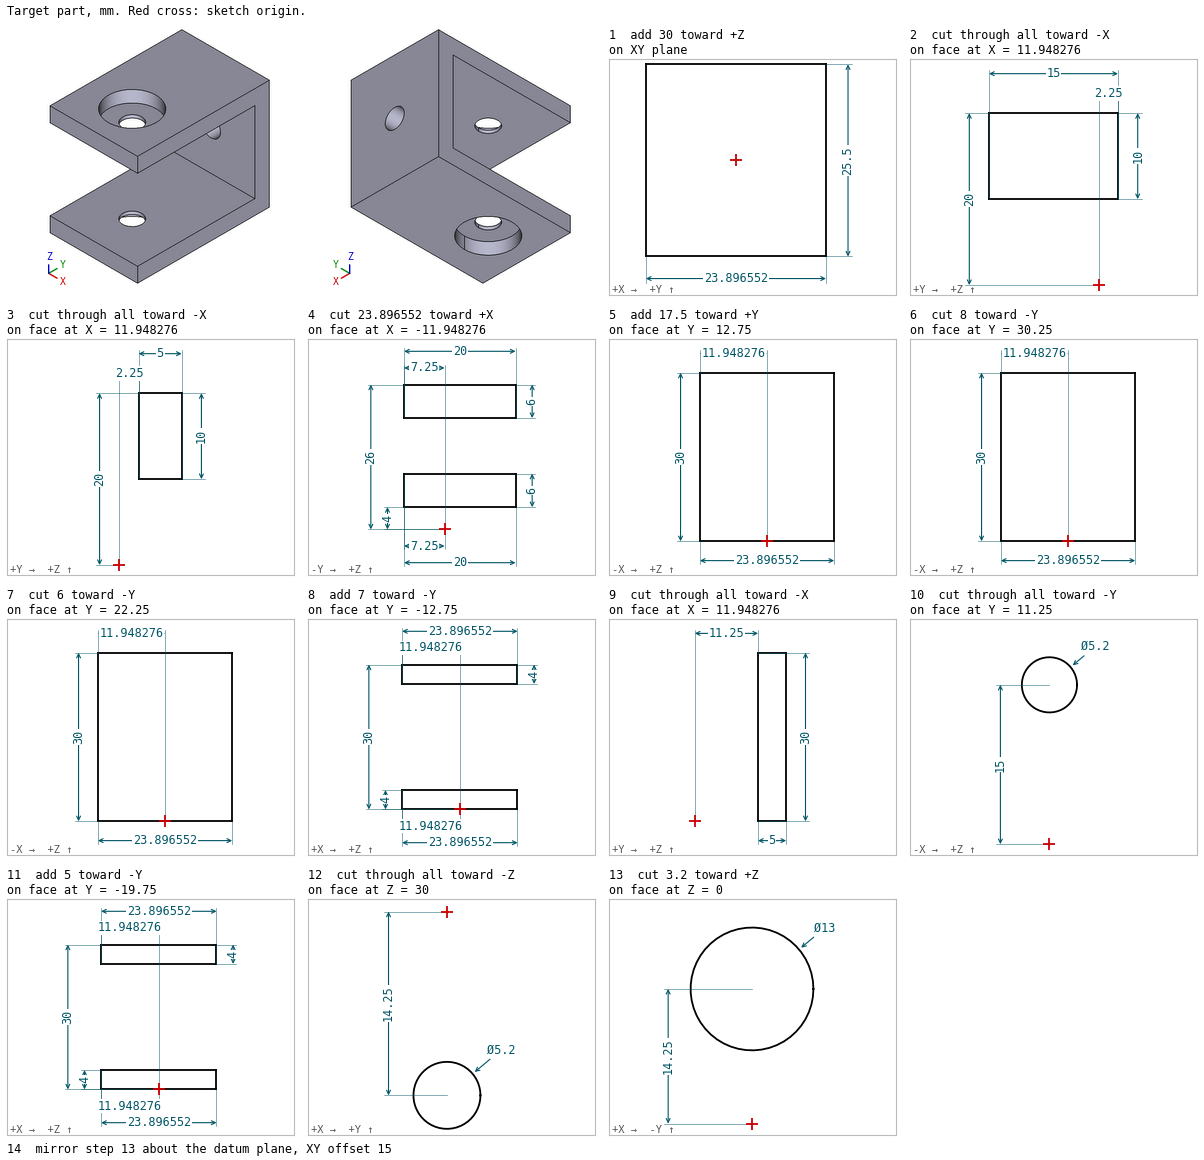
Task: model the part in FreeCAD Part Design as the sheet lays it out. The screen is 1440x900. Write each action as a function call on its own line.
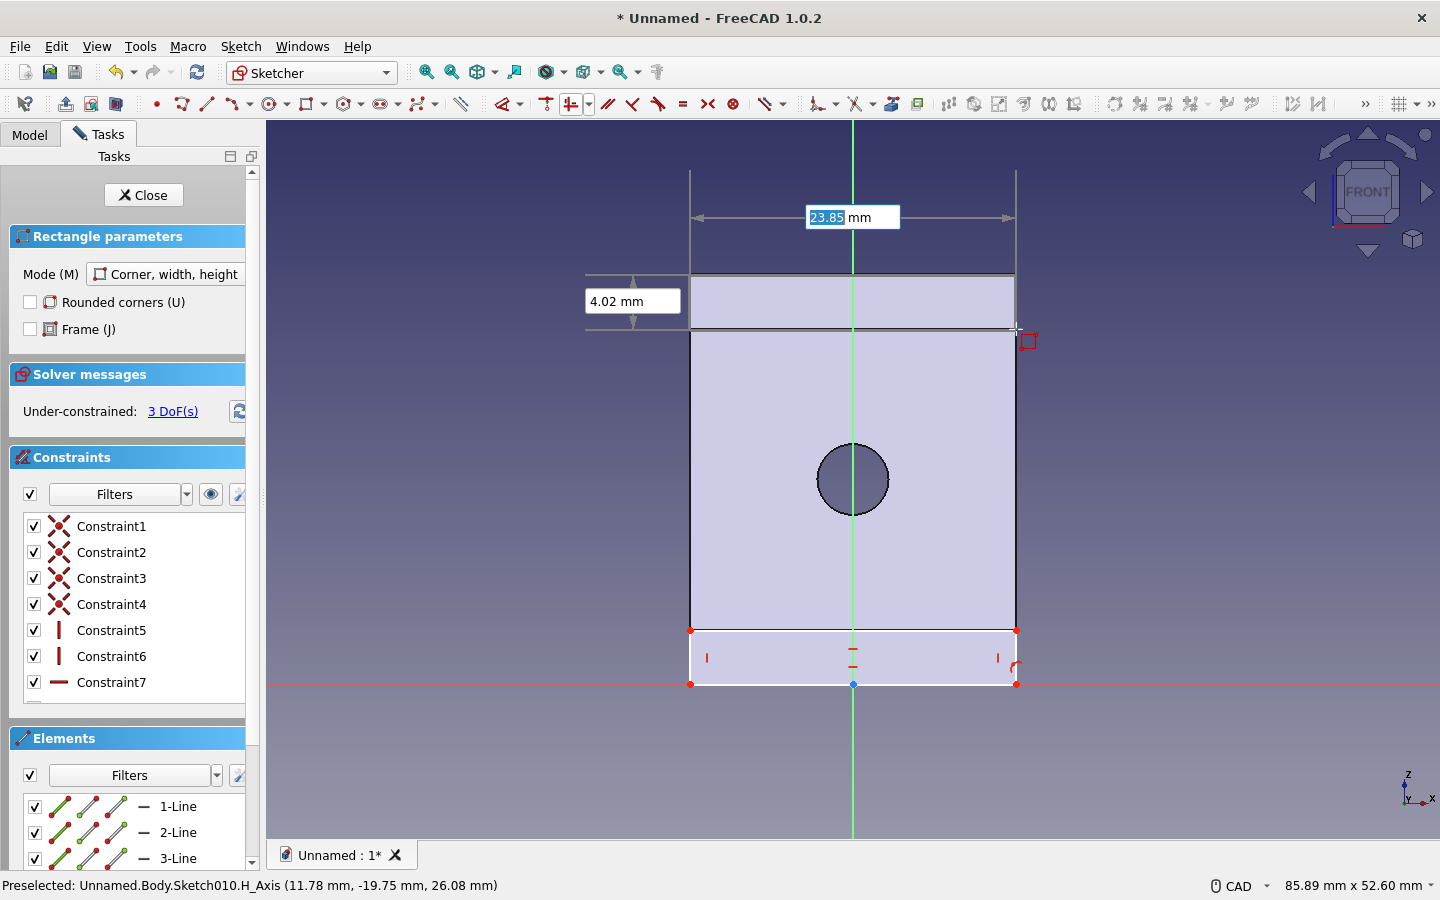
text(23.896552)
key(Tab)
text(4)
key(Return)
key(Escape)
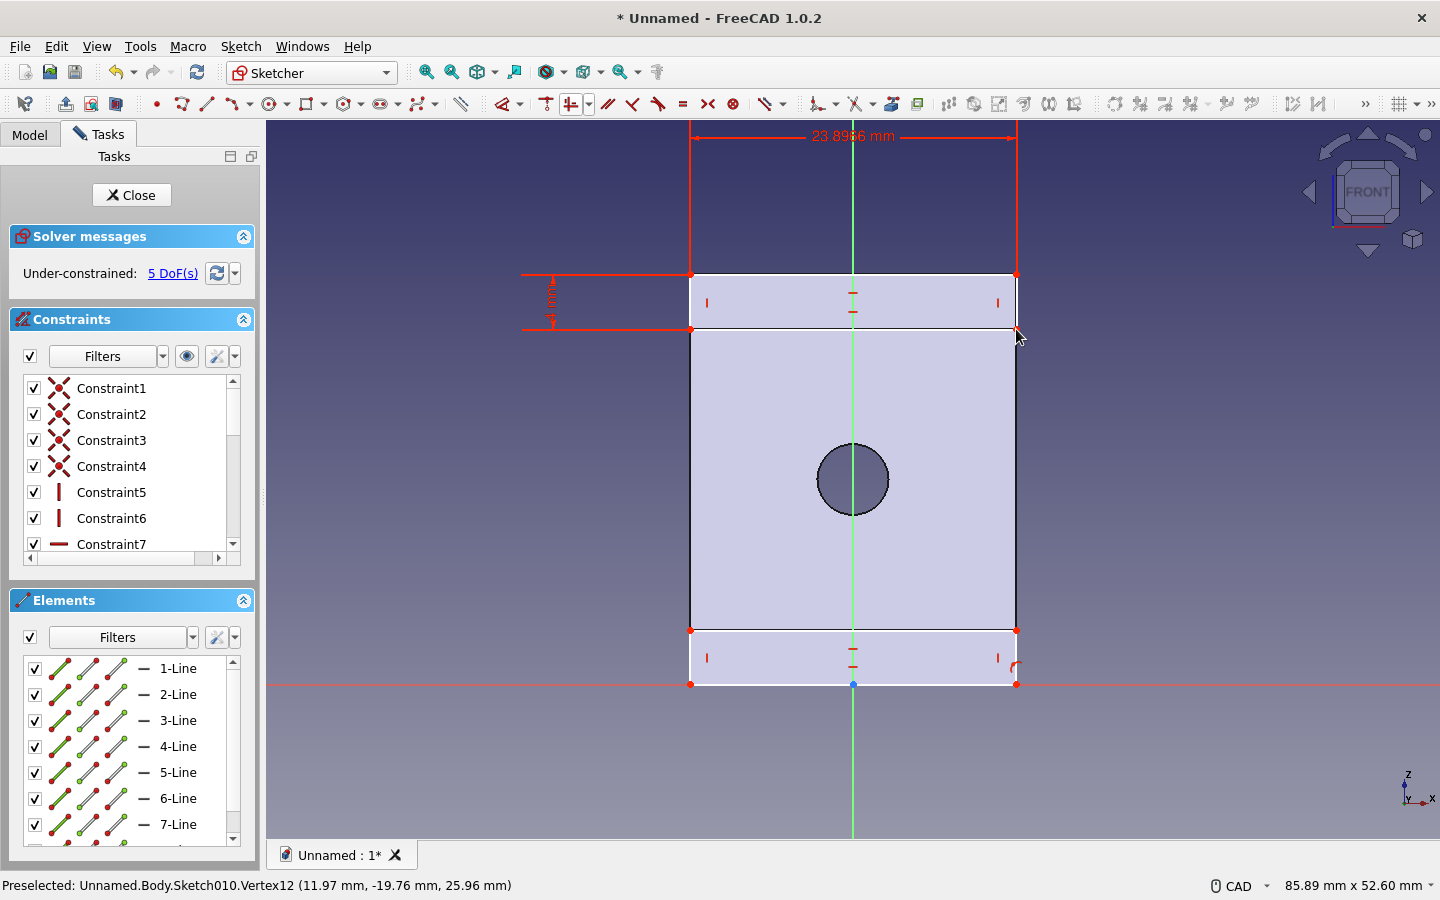
key(d)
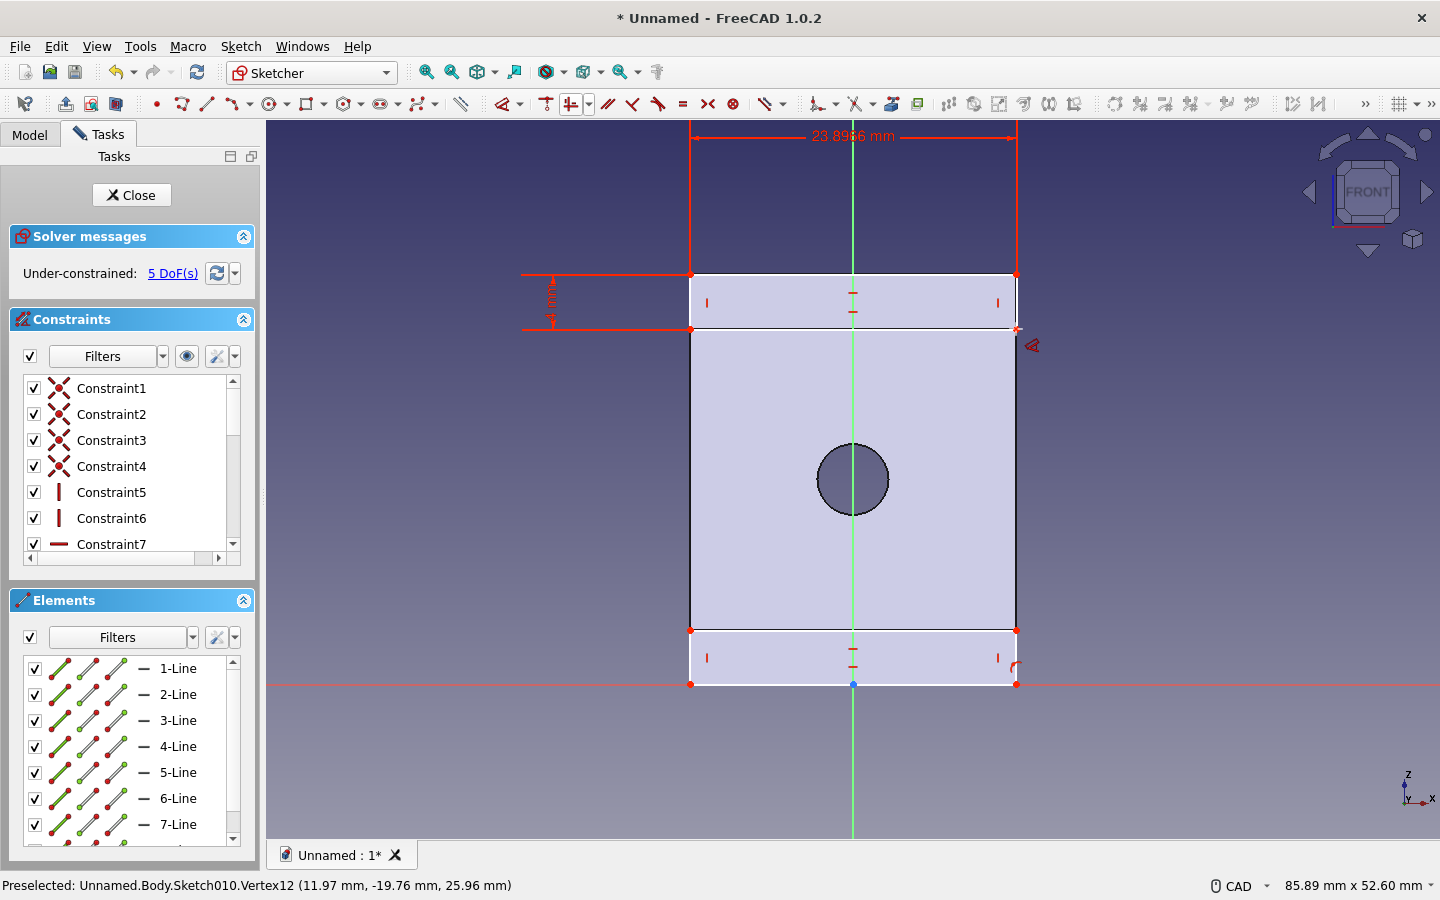
click(690, 647)
click(656, 658)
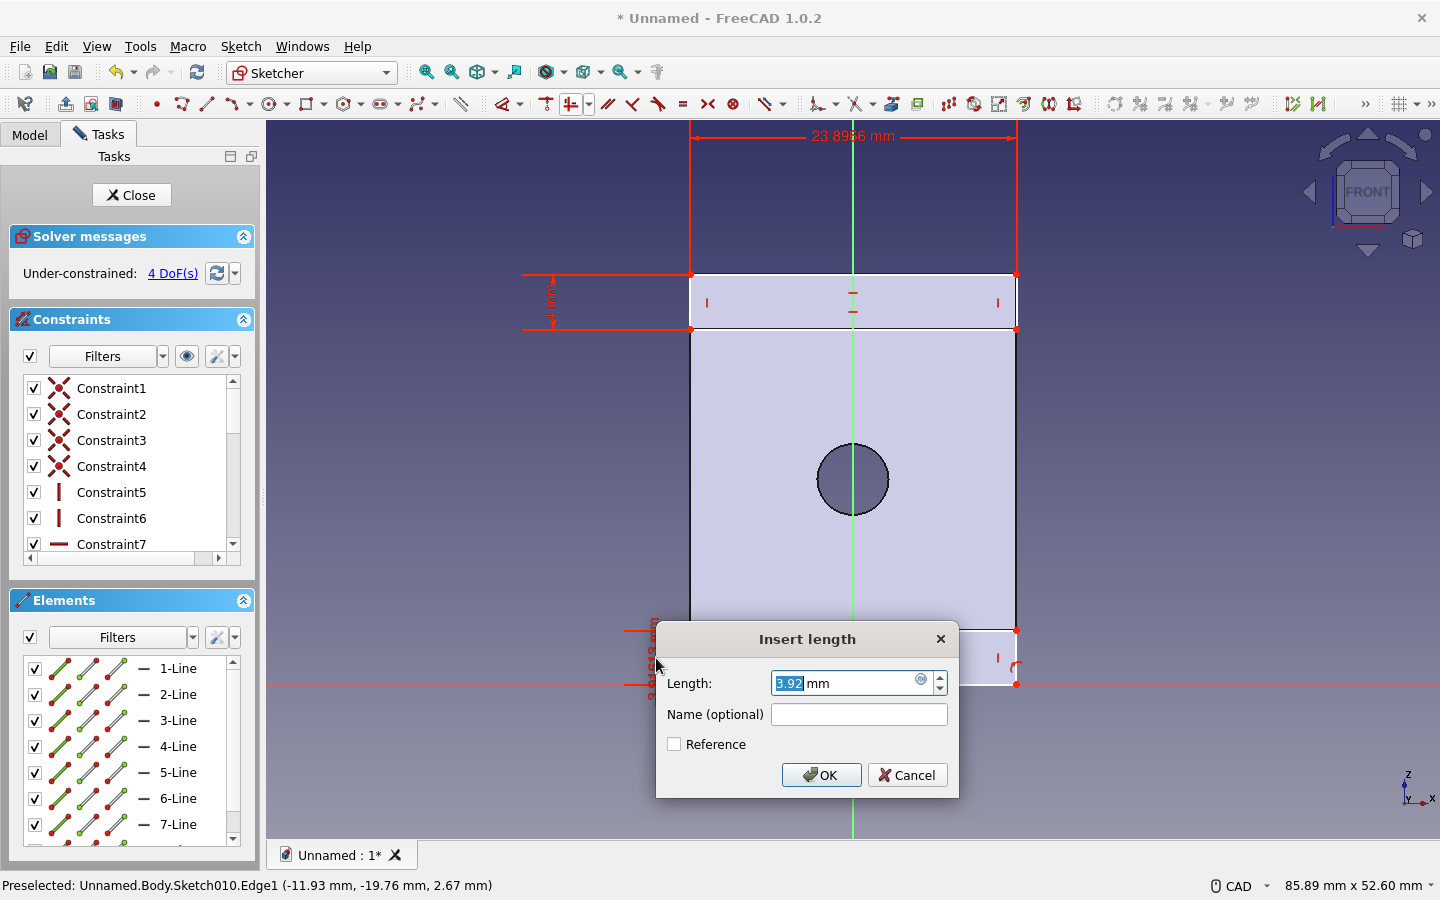
text(4)
key(Return)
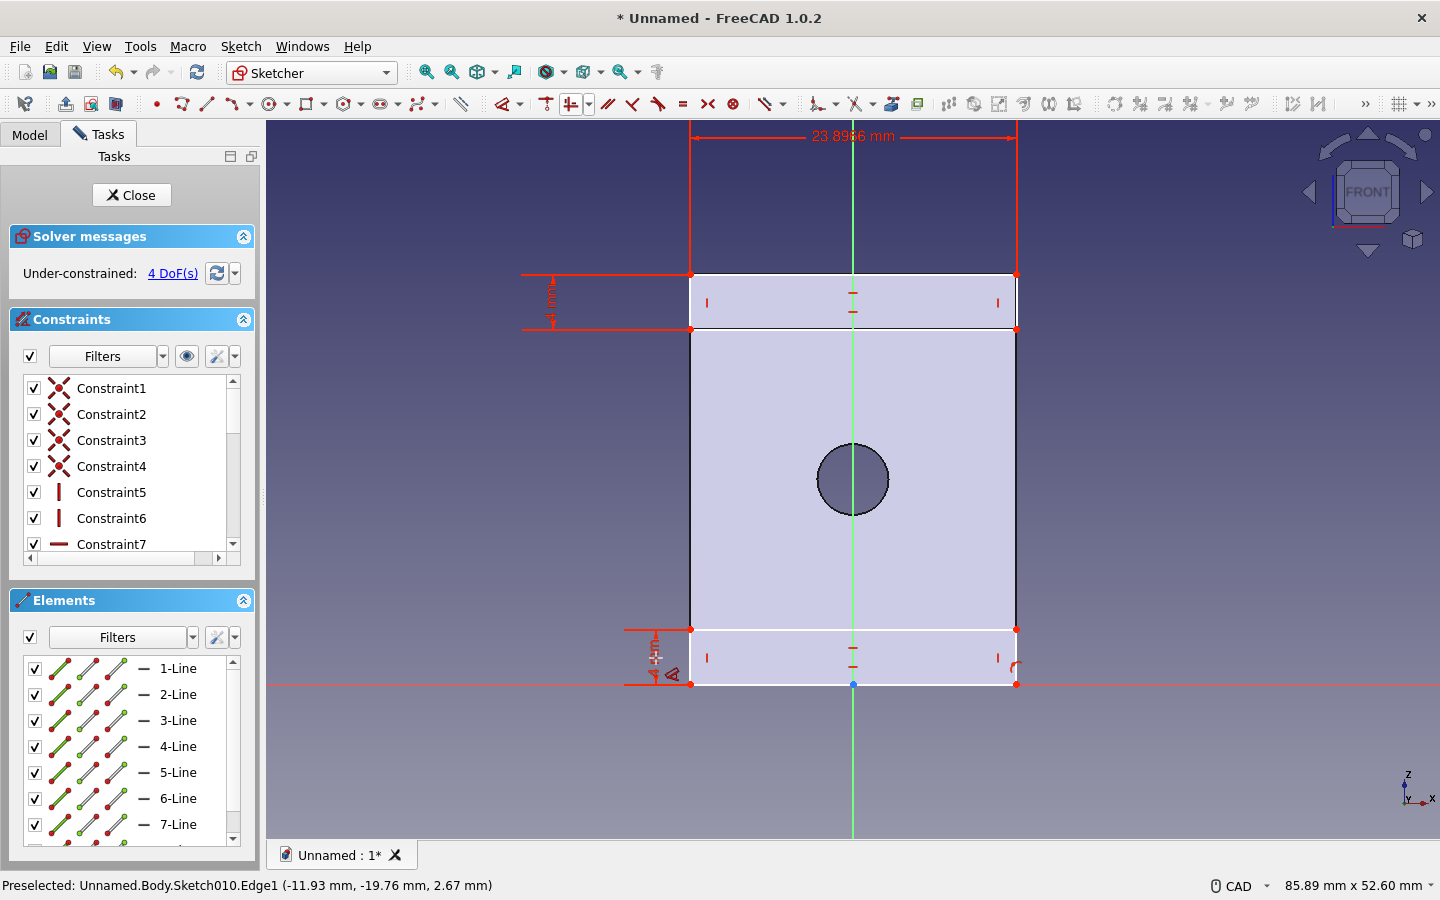
click(690, 275)
click(656, 480)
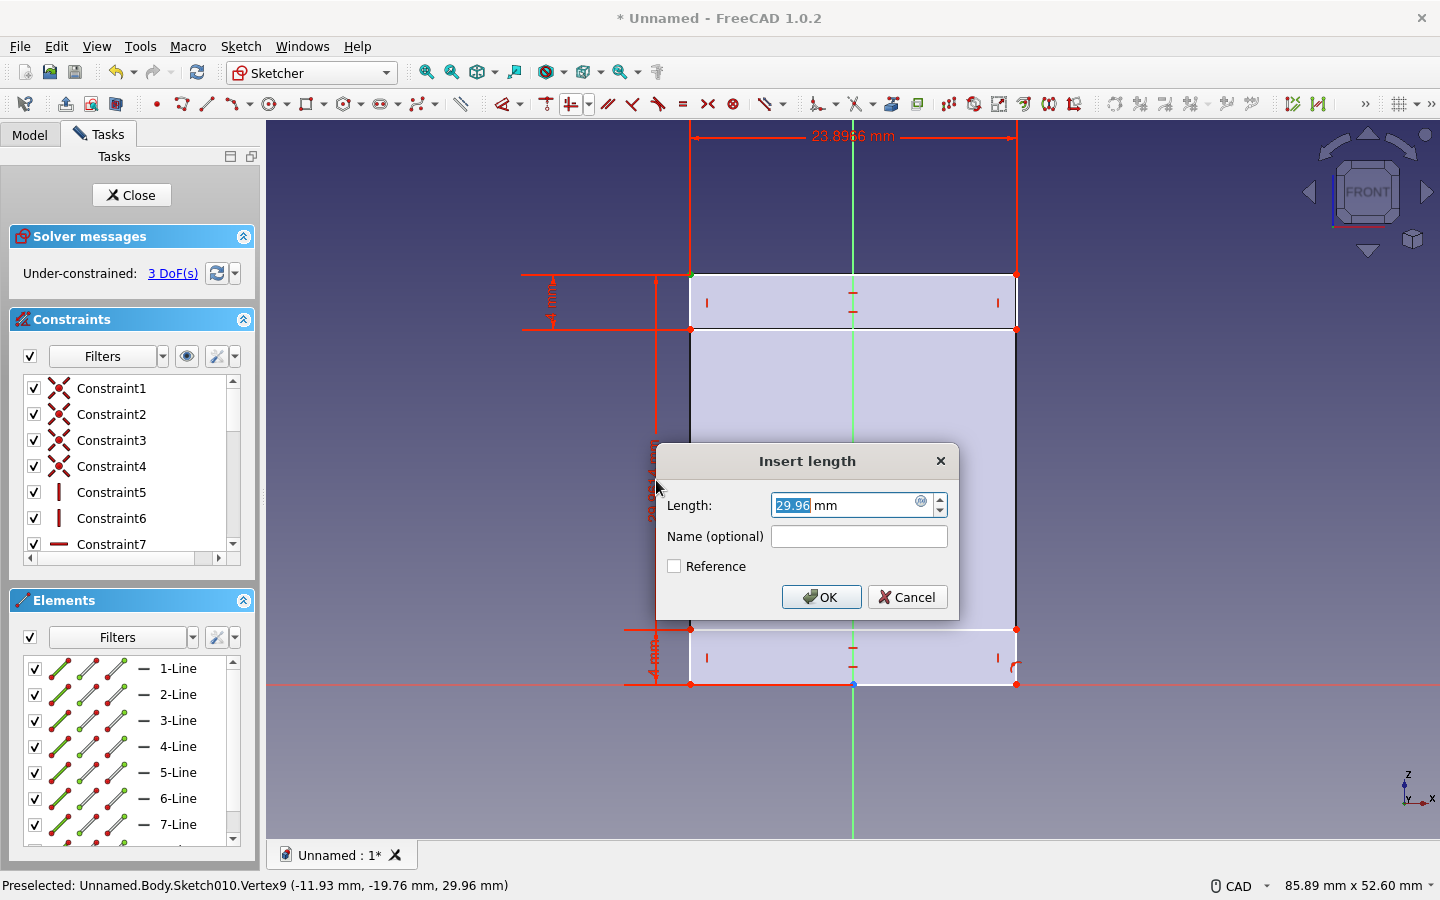
text(30)
key(Return)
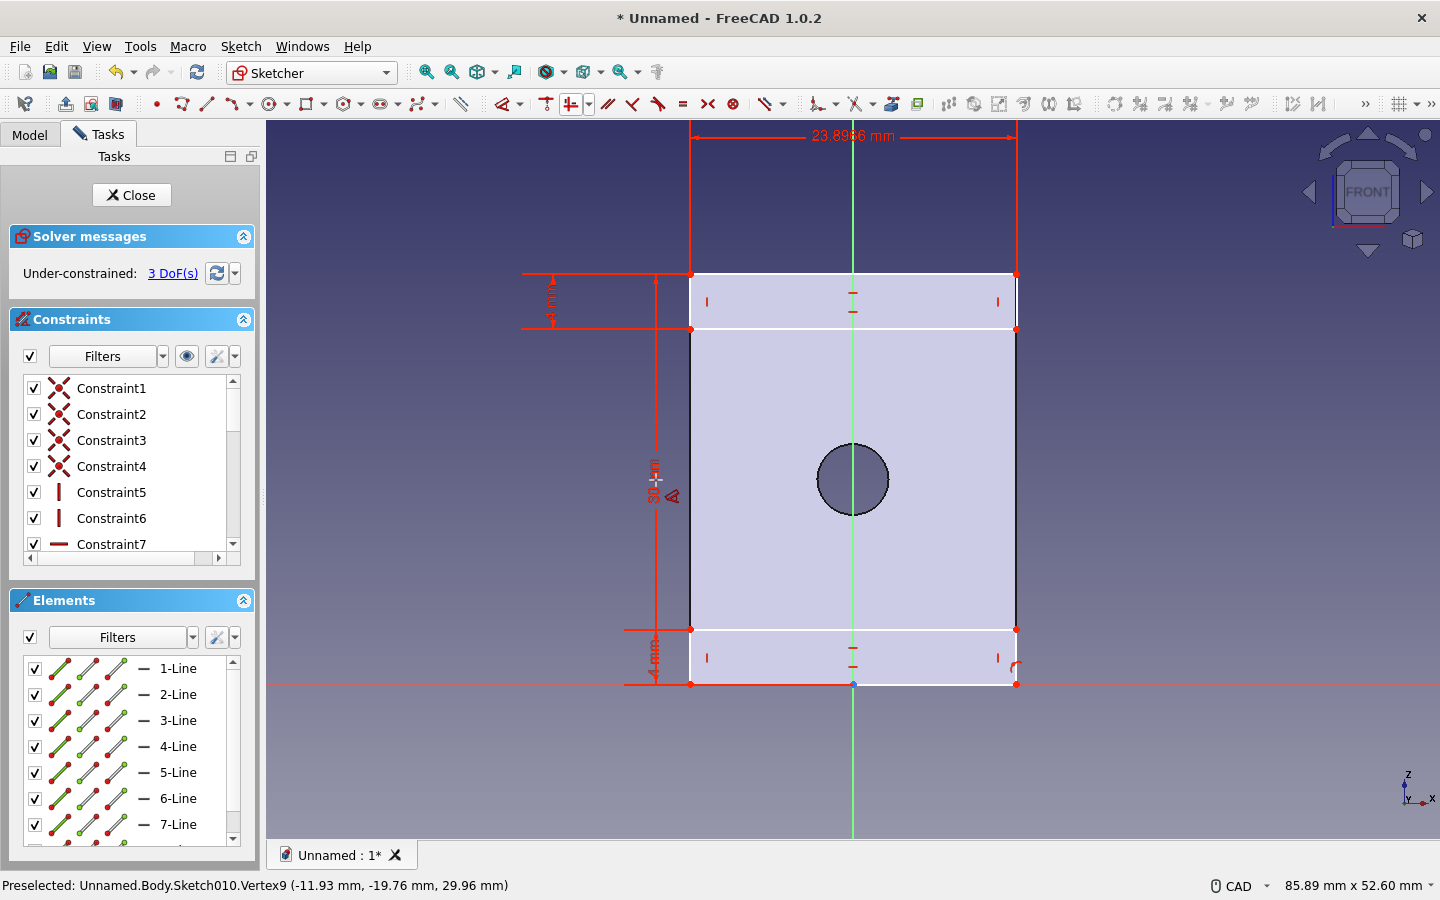
click(788, 685)
click(778, 719)